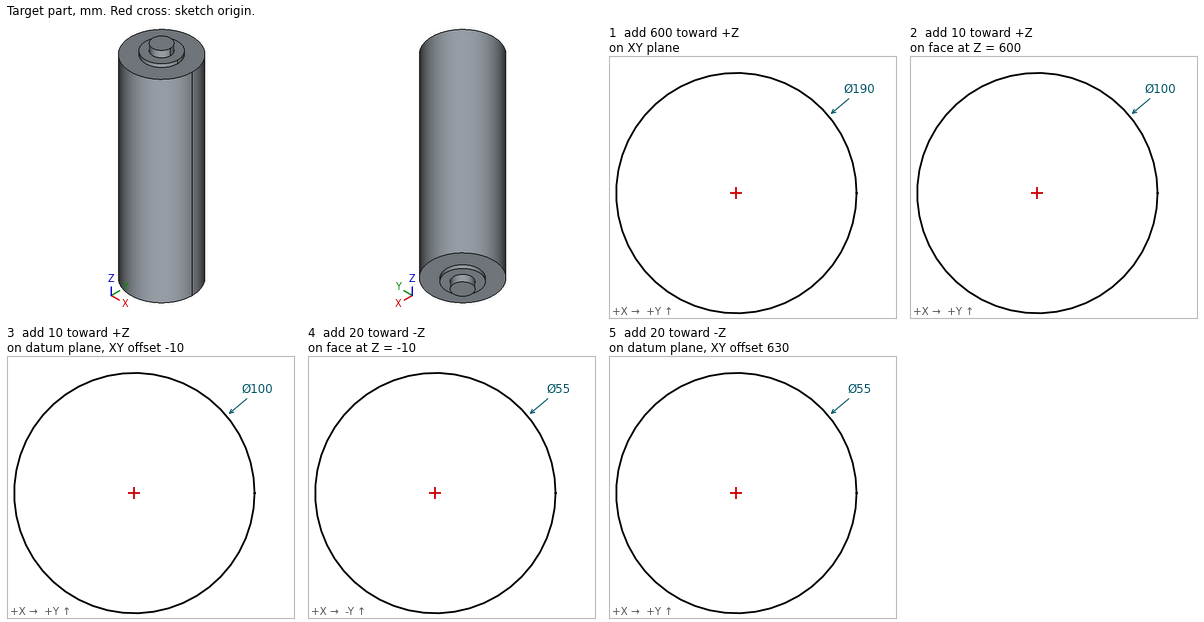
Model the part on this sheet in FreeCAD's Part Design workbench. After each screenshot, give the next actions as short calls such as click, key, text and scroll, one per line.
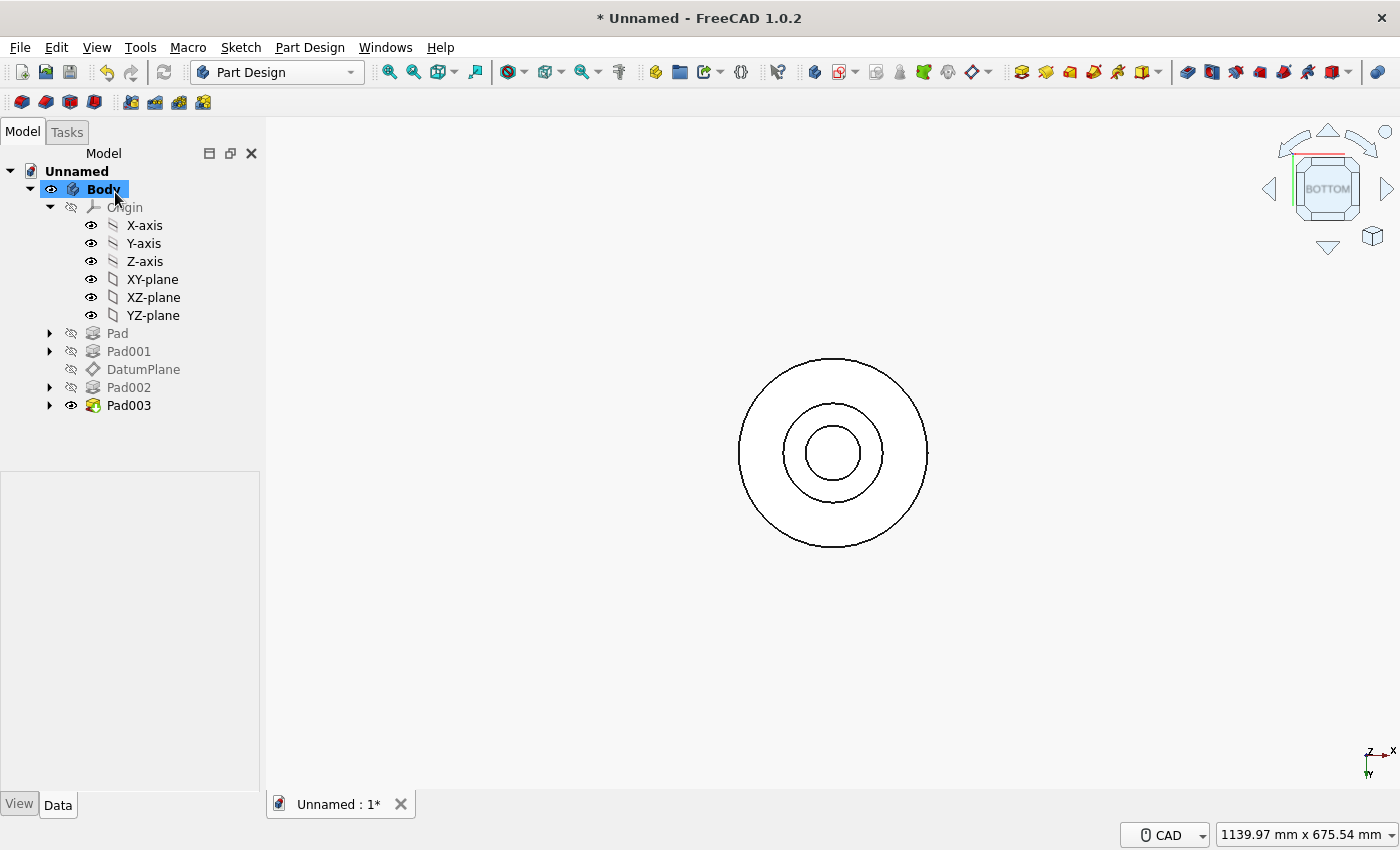
click(390, 72)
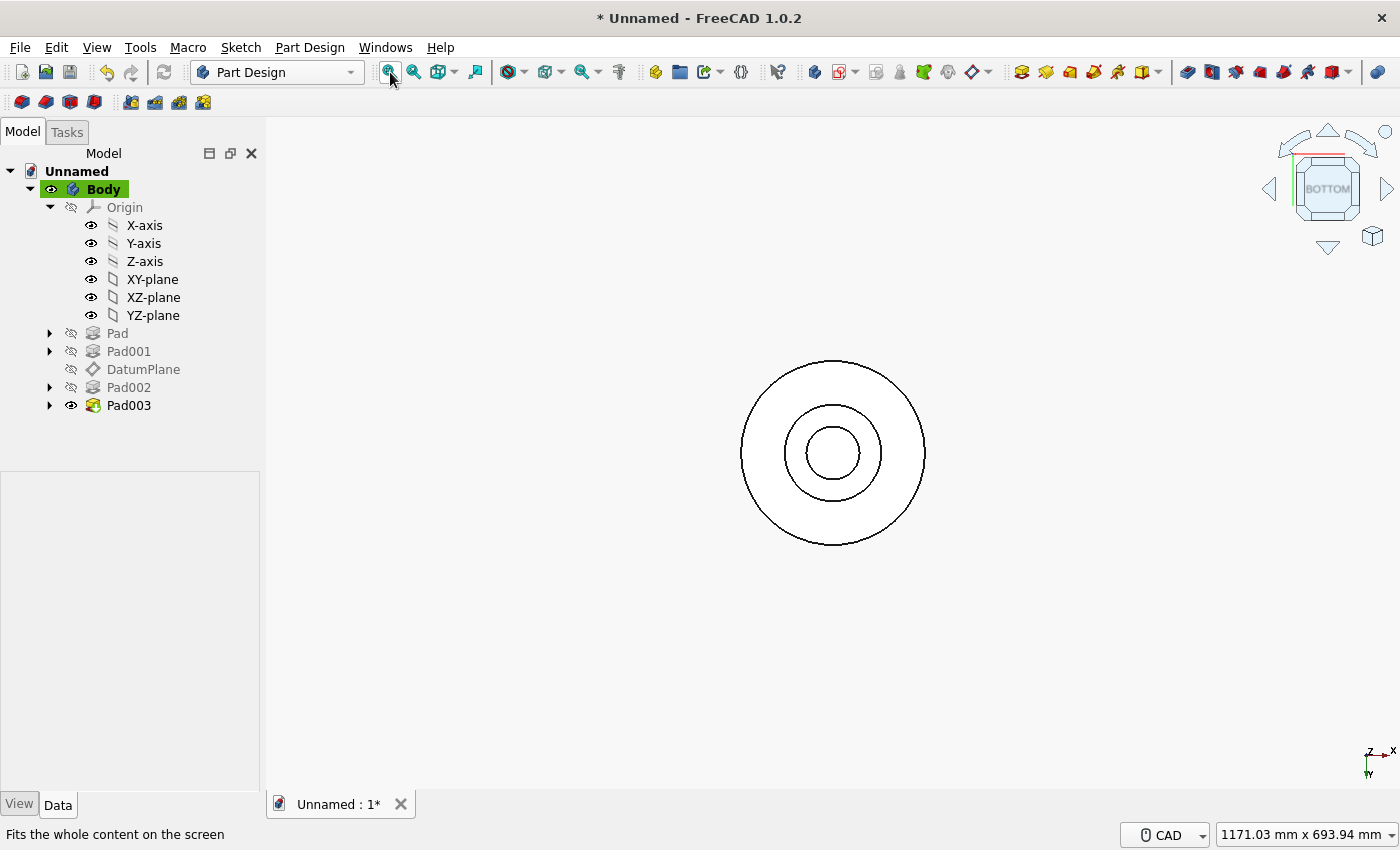
click(136, 279)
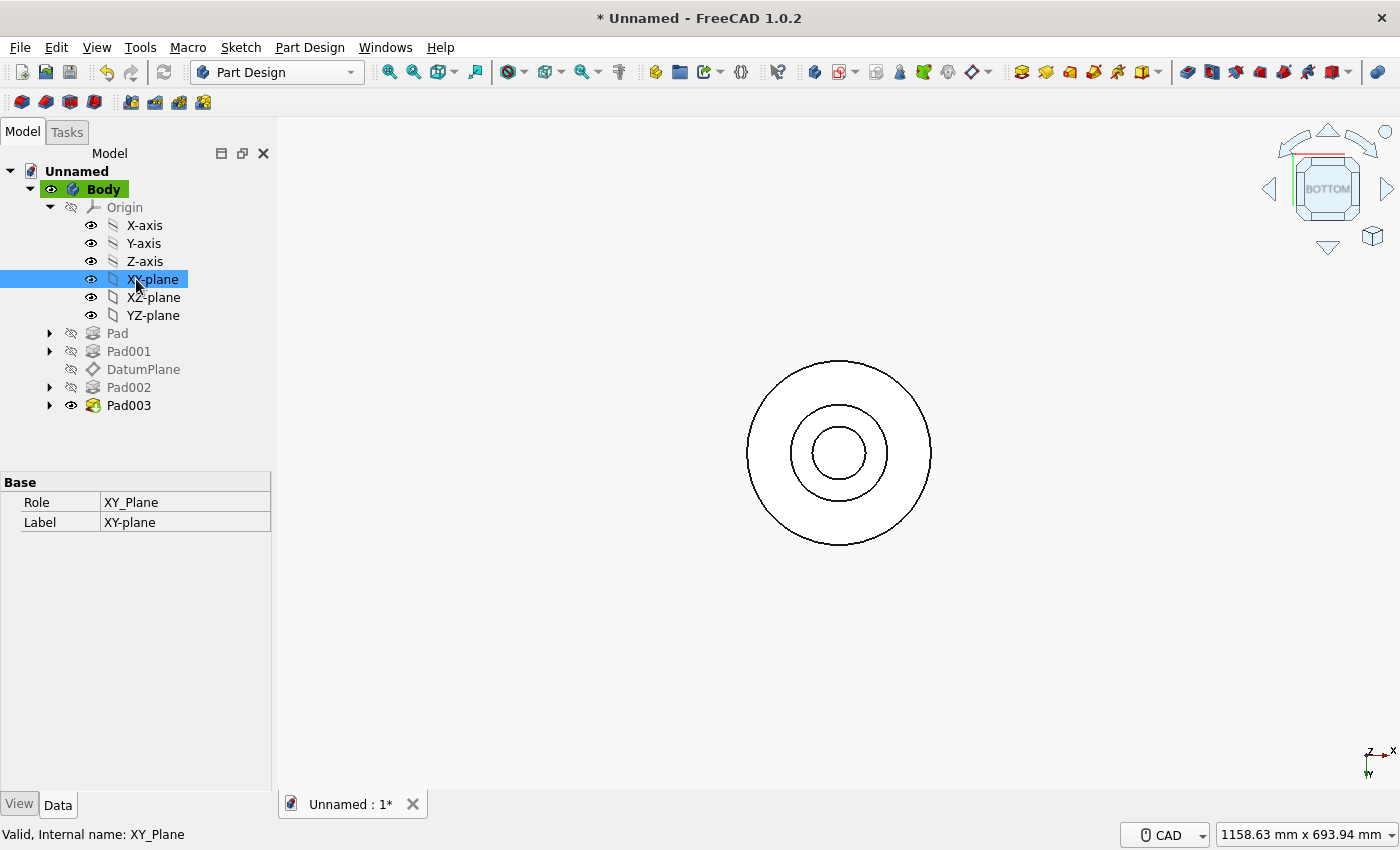
click(972, 72)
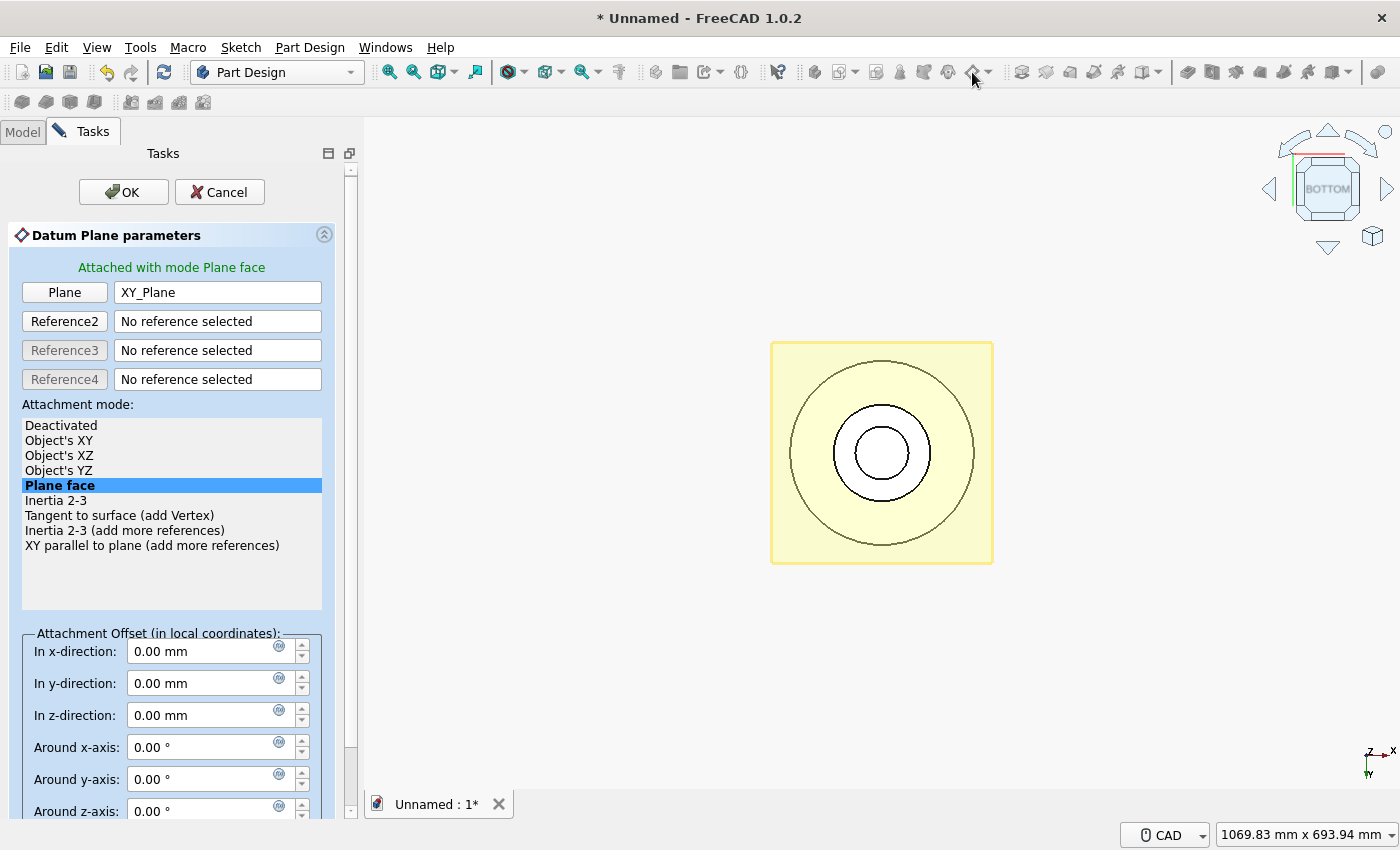
triple_click(210, 715)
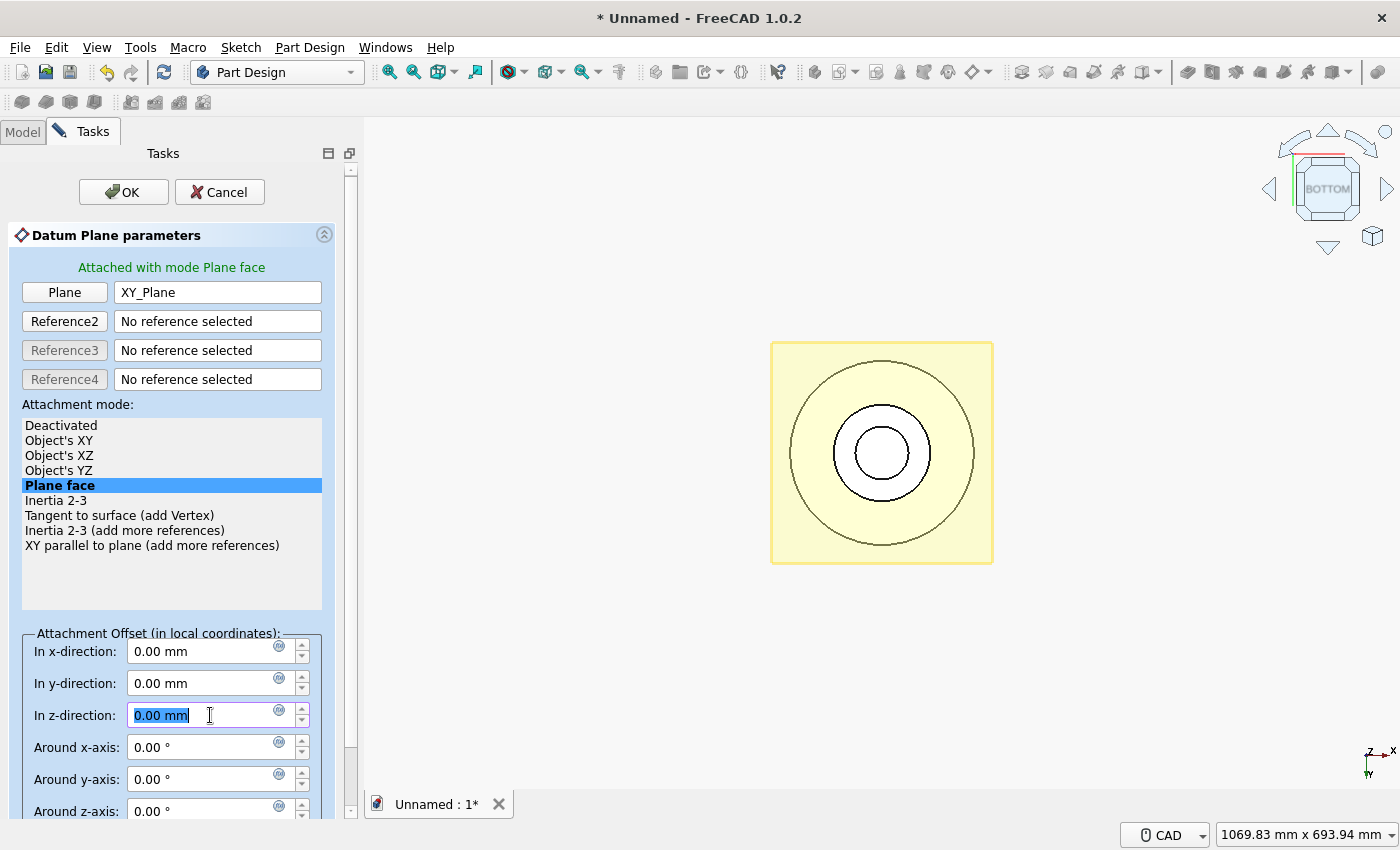
text(630)
key(Tab)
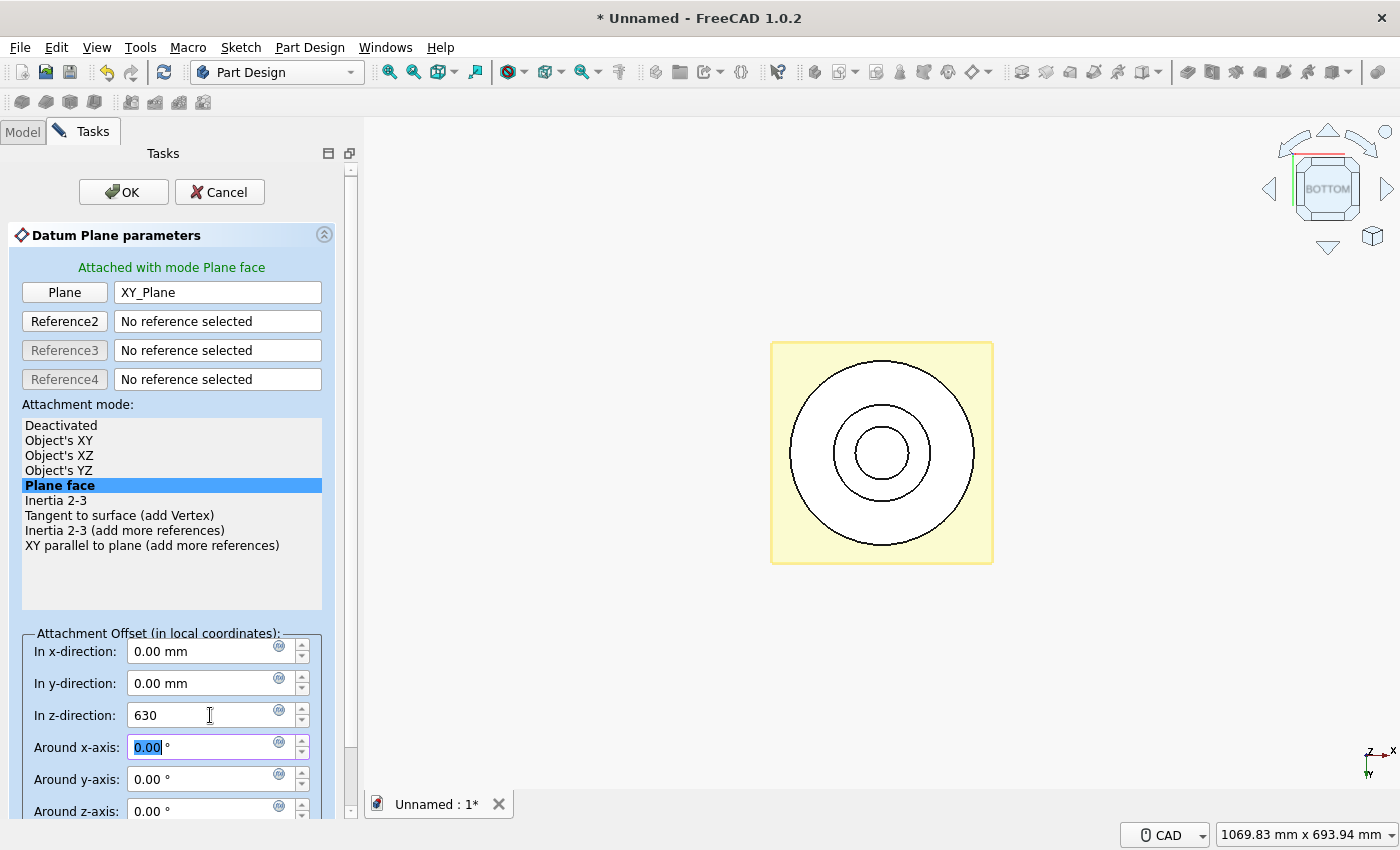
click(124, 192)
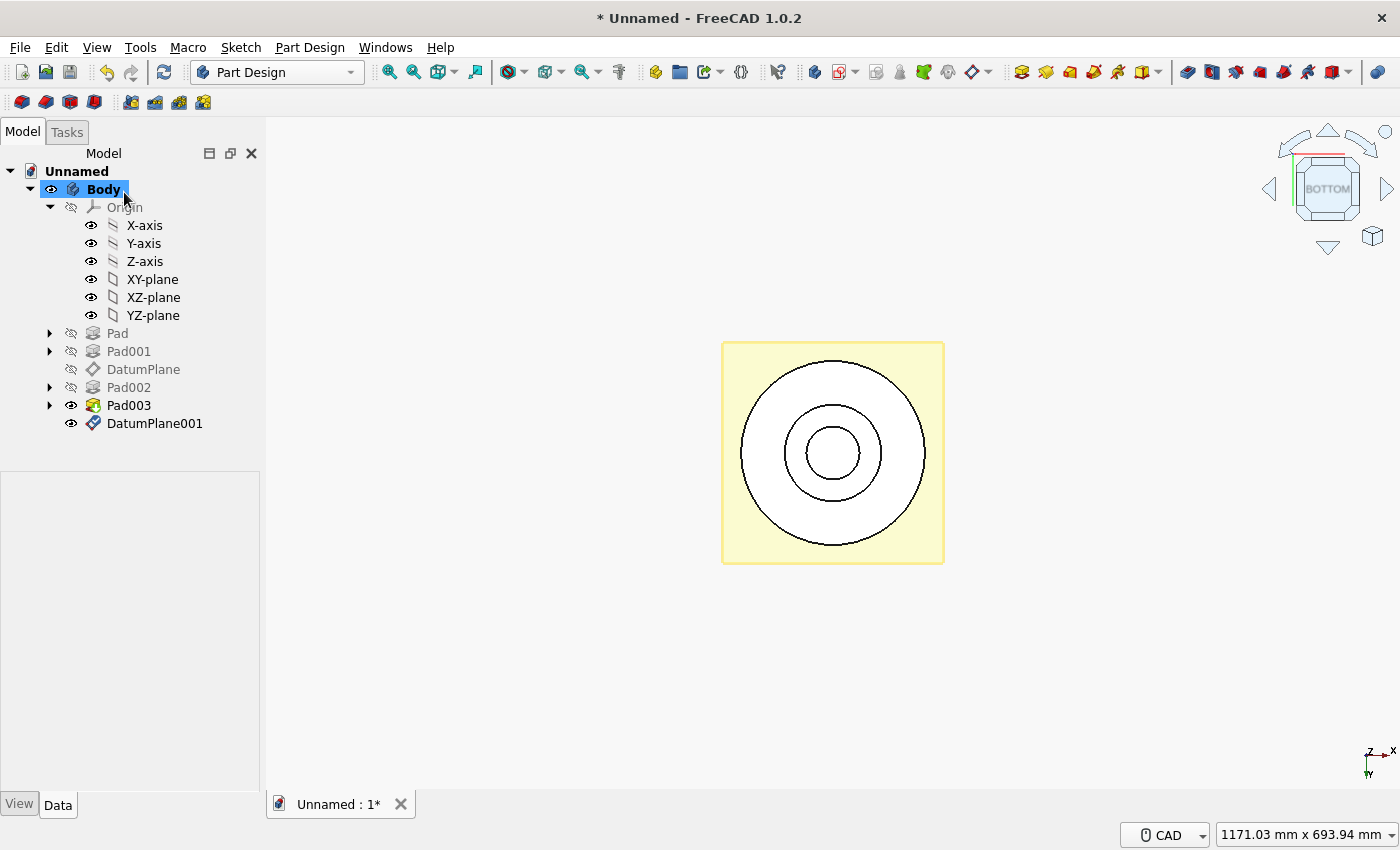
click(116, 423)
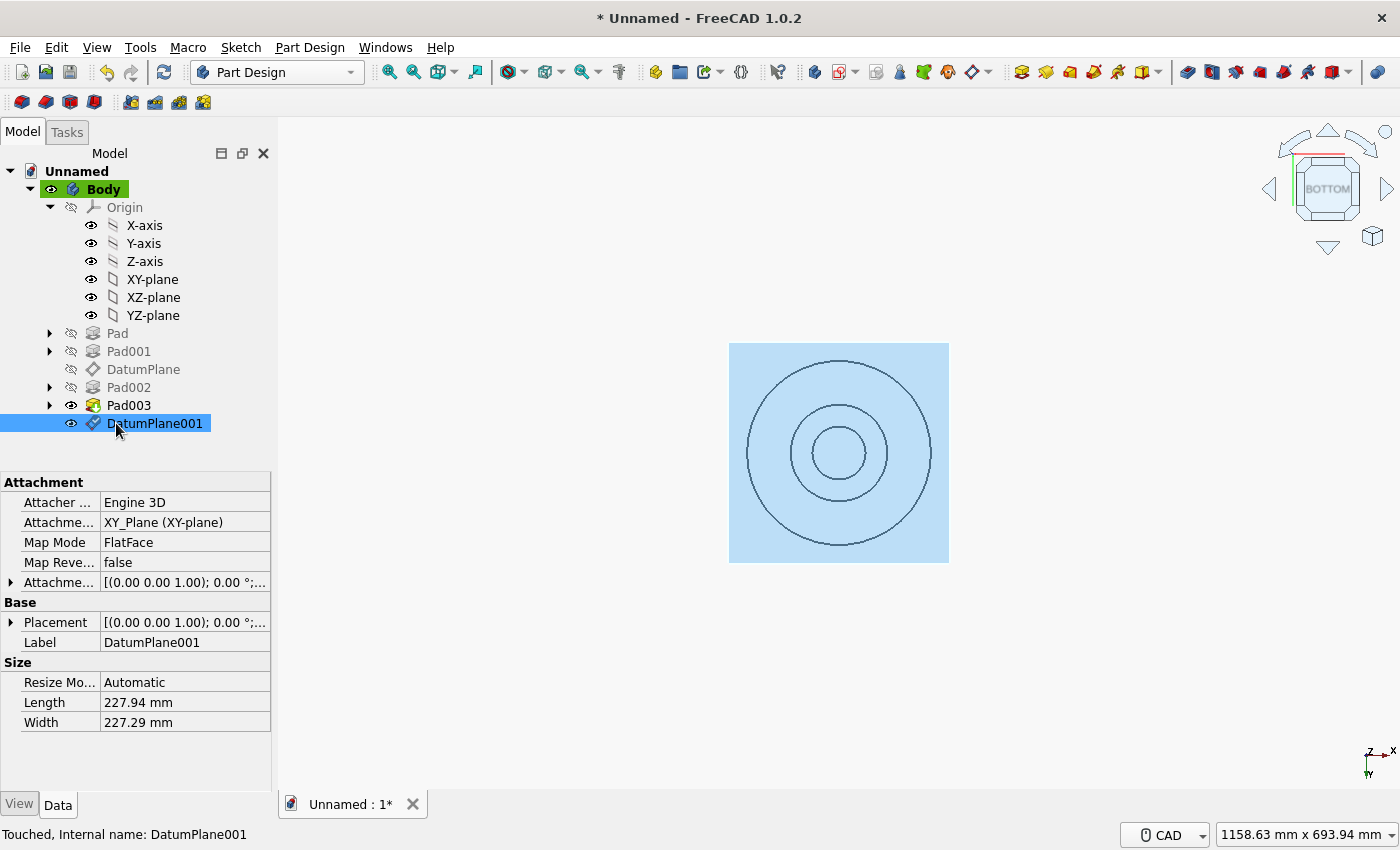
click(840, 72)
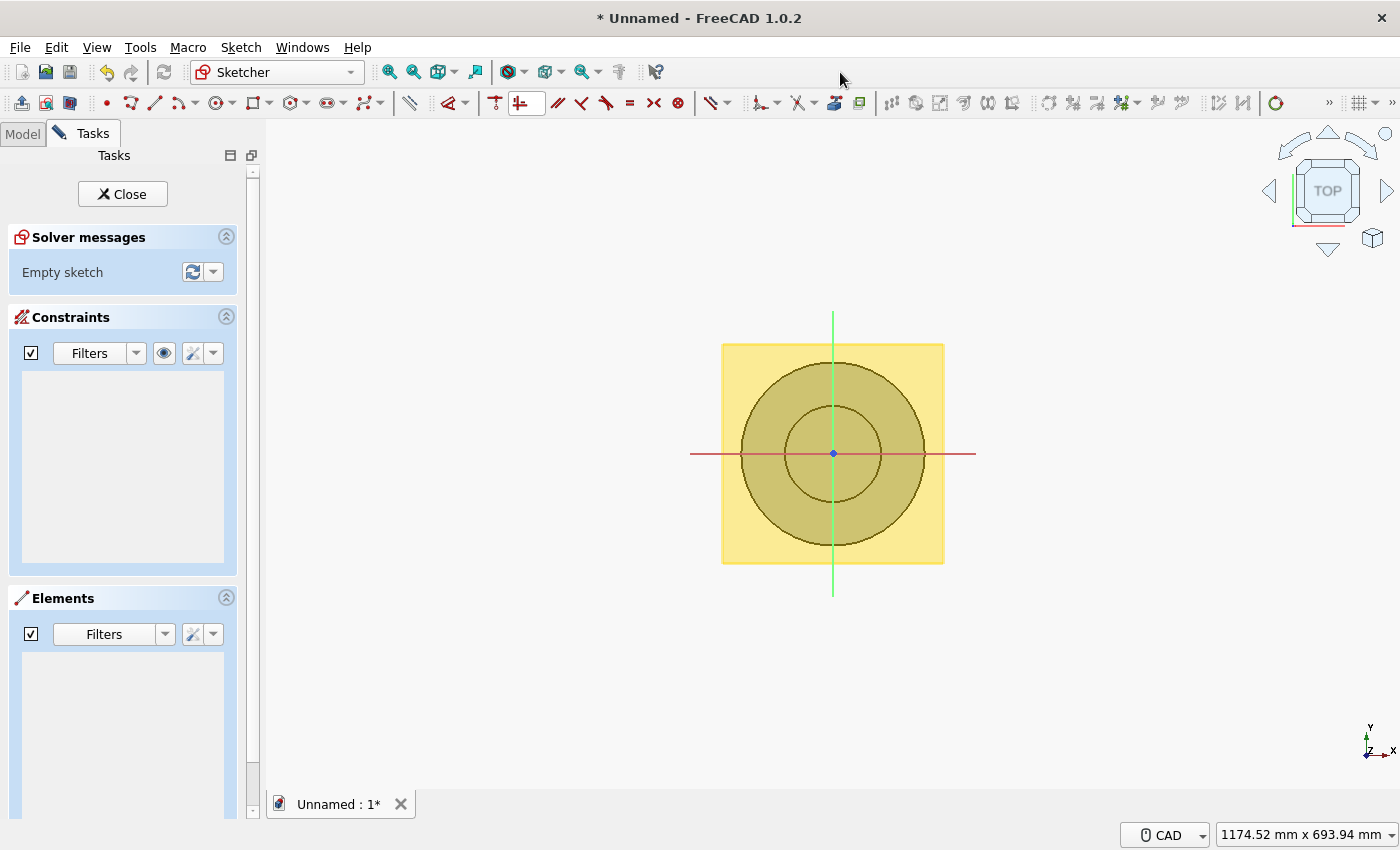
scroll(844, 454, up, 10)